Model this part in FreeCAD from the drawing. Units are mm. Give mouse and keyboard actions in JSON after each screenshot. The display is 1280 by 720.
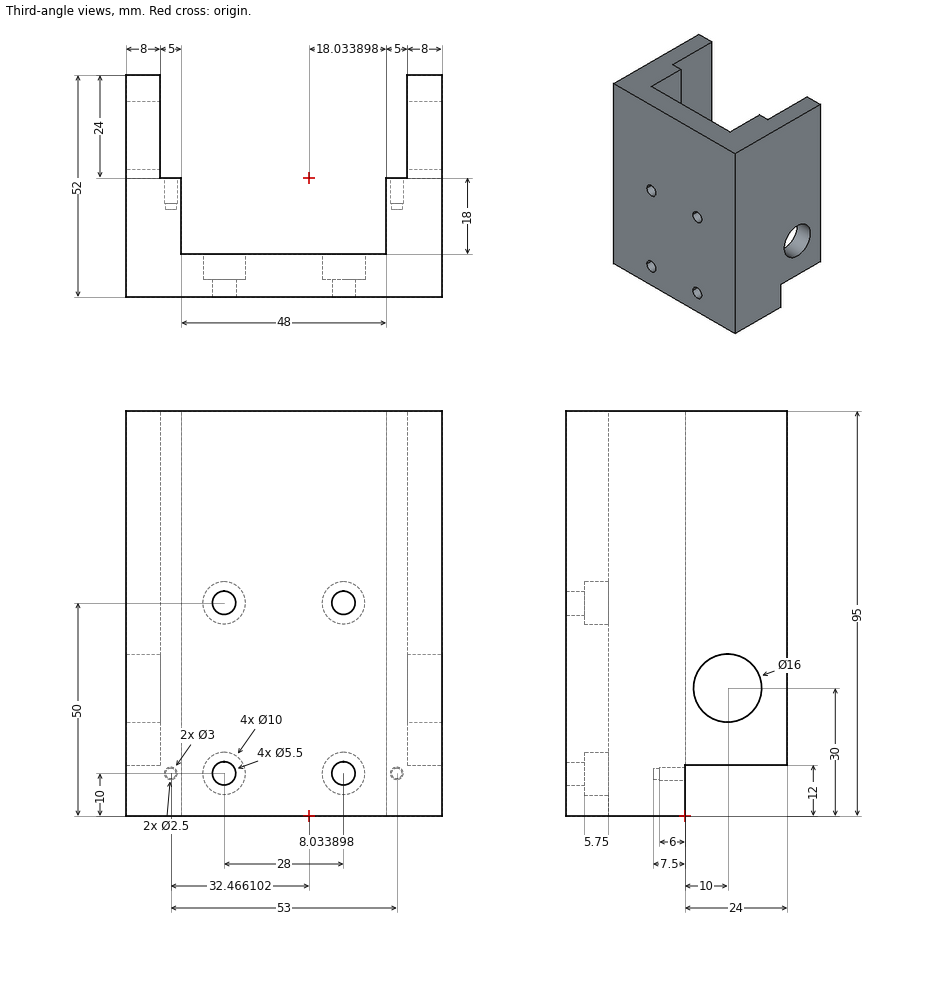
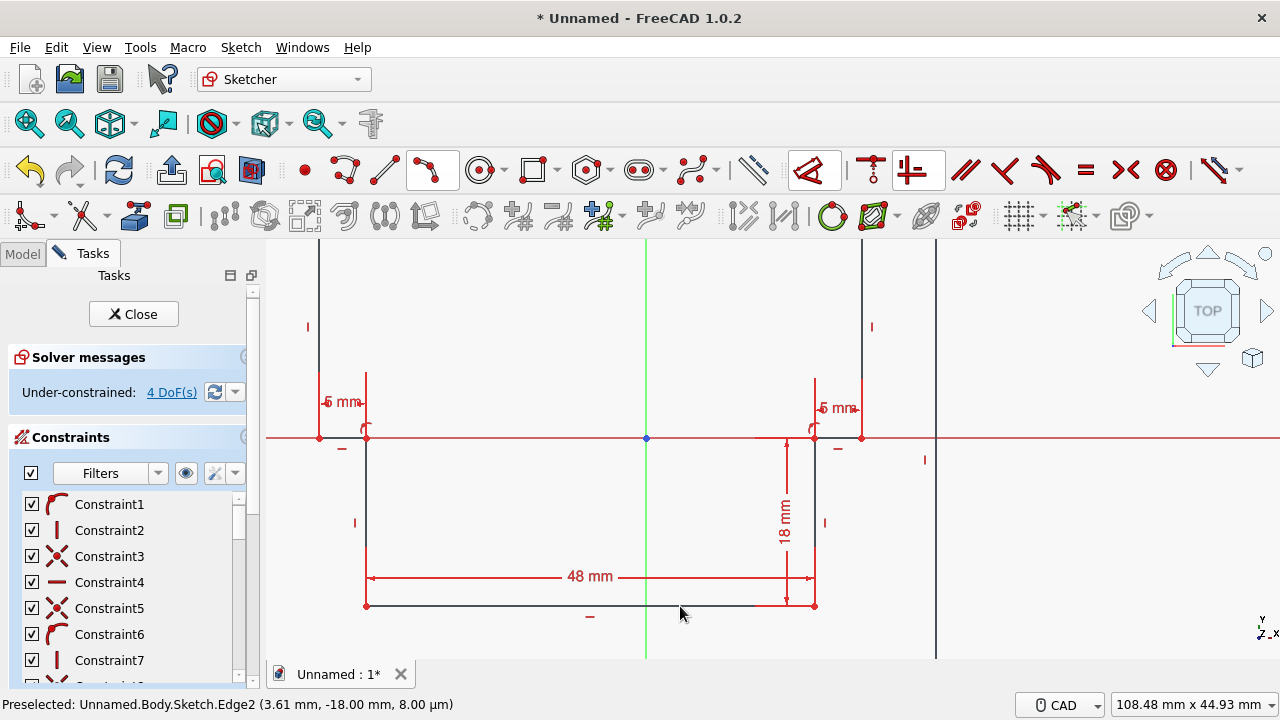
{"action": "left_click", "coordinate": [319, 371]}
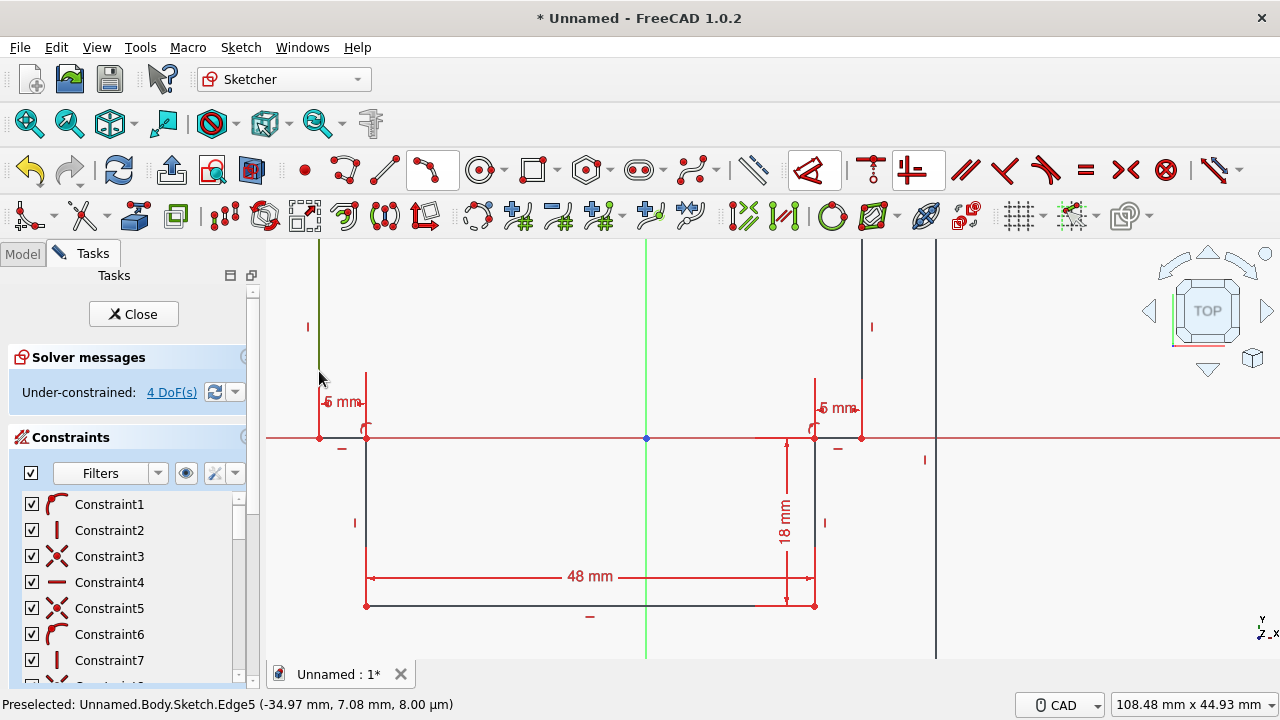
{"action": "key", "text": "i"}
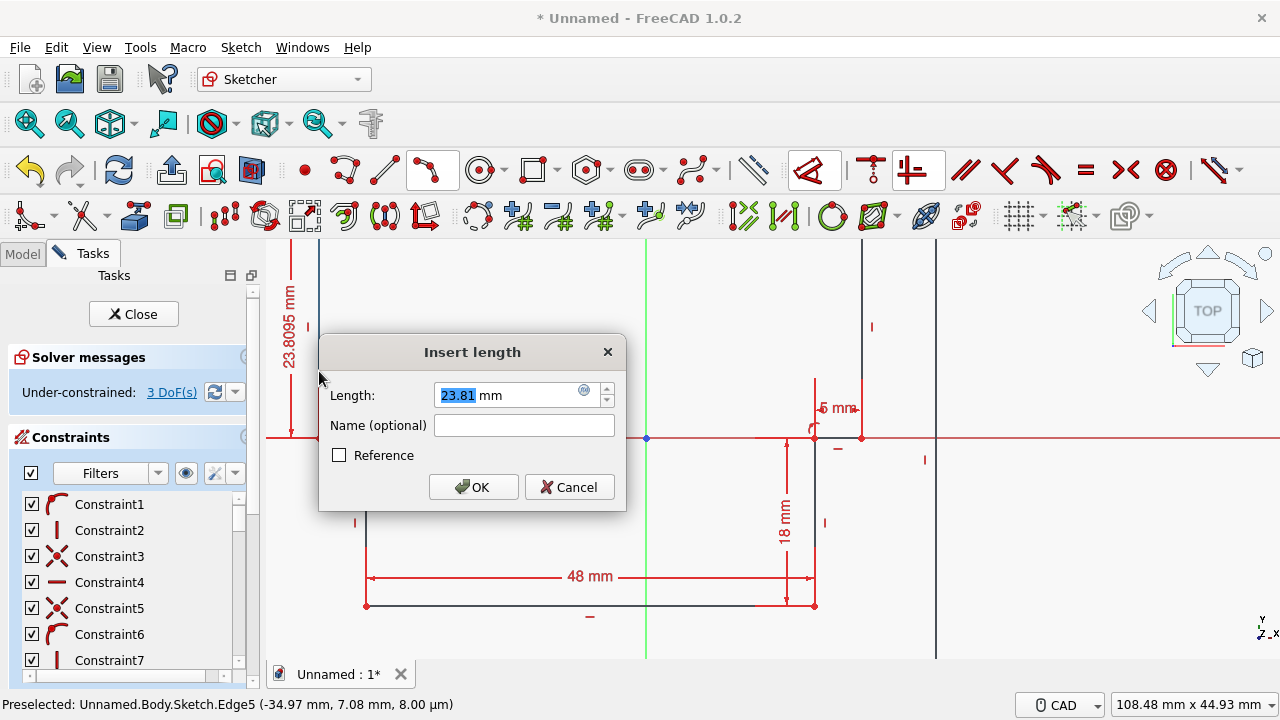
{"action": "type", "text": "24"}
{"action": "key", "text": "Return"}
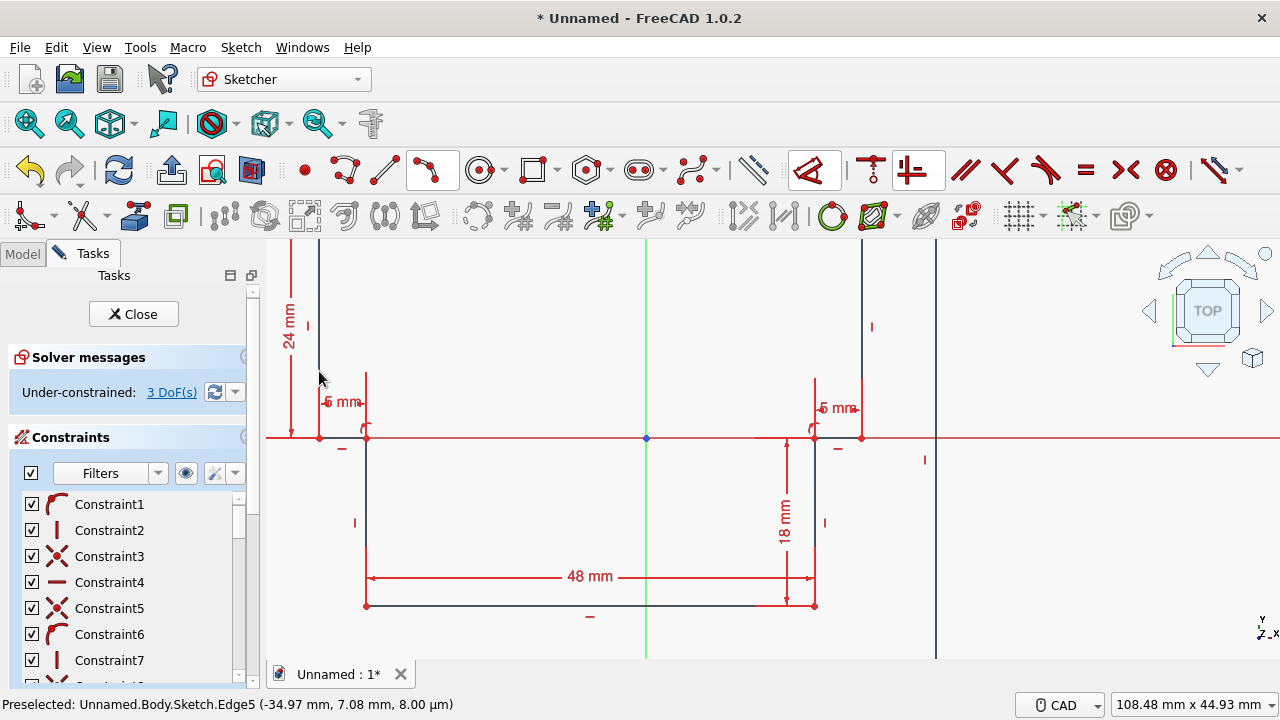
{"action": "scroll", "coordinate": [843, 439], "scroll_direction": "down", "scroll_amount": 3}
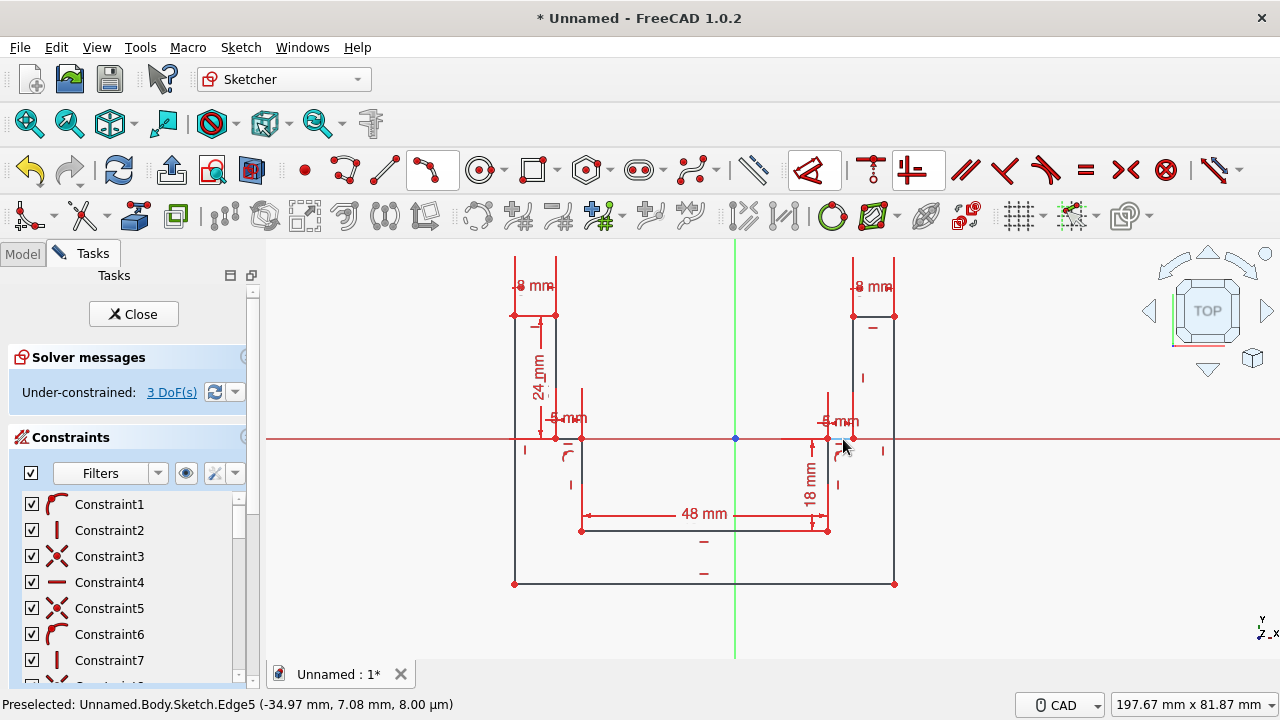
{"action": "left_click", "coordinate": [515, 396]}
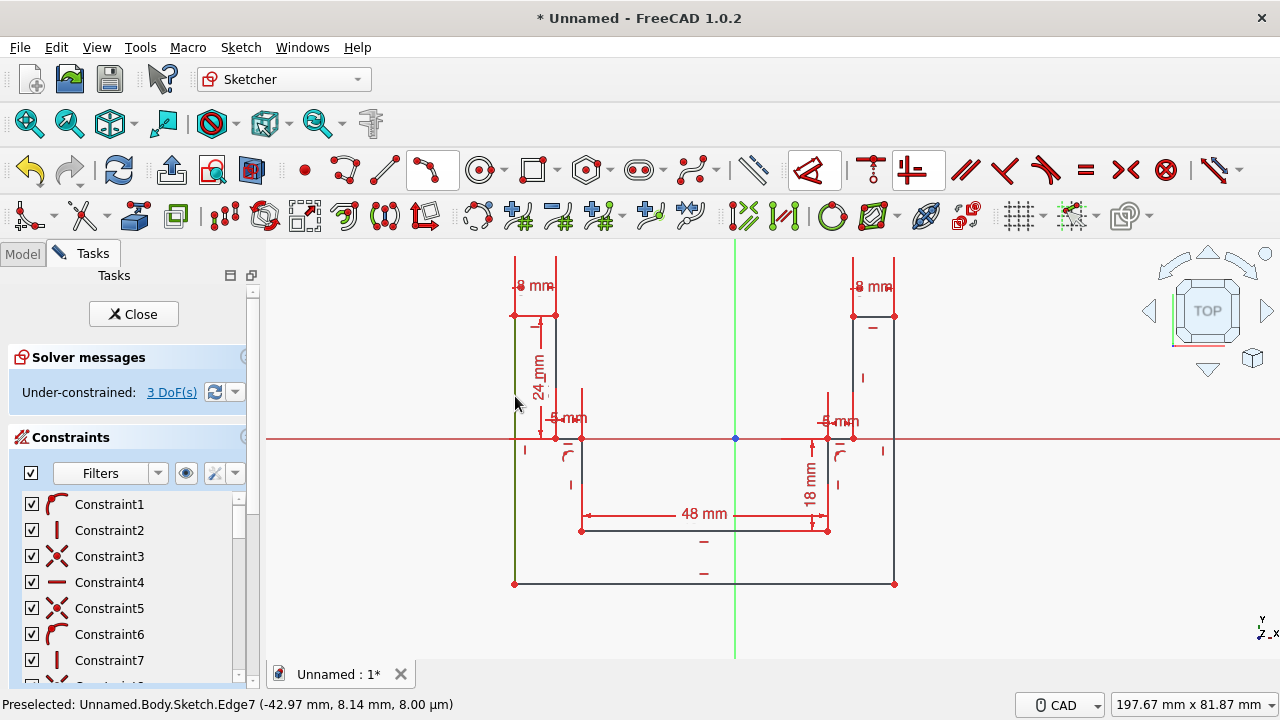
{"action": "key", "text": "i"}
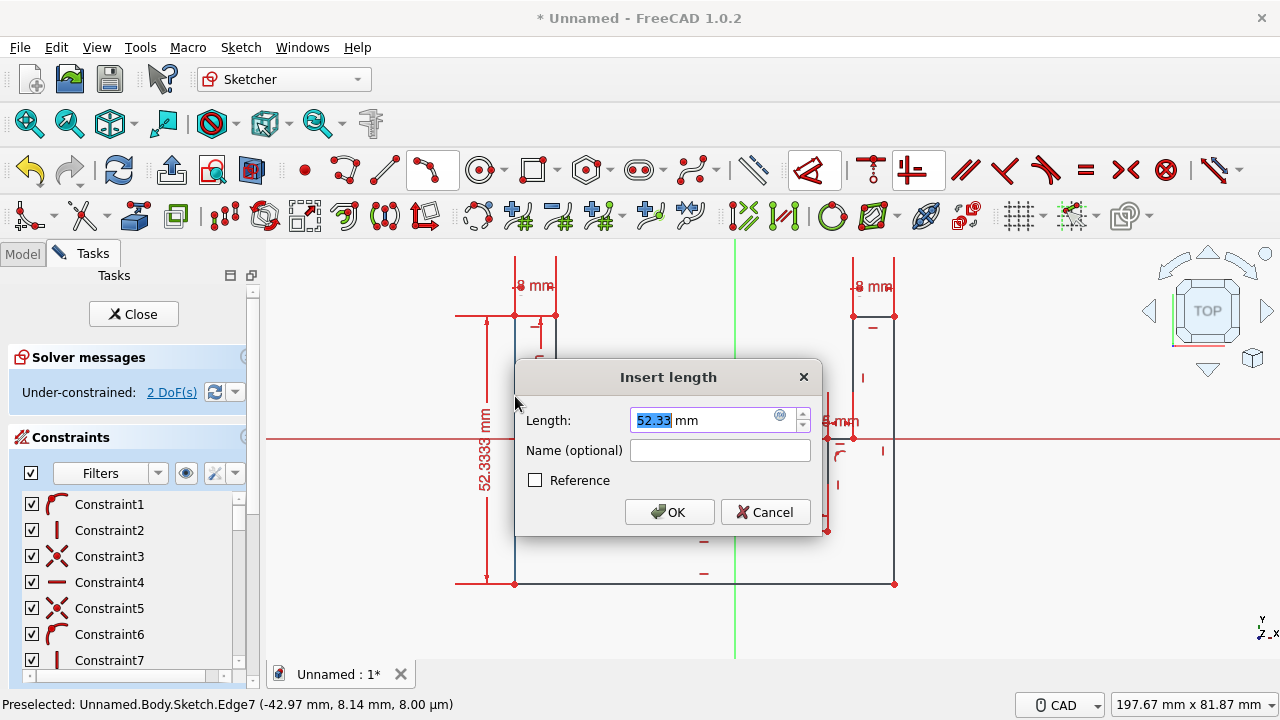
{"action": "type", "text": "52"}
{"action": "key", "text": "Return"}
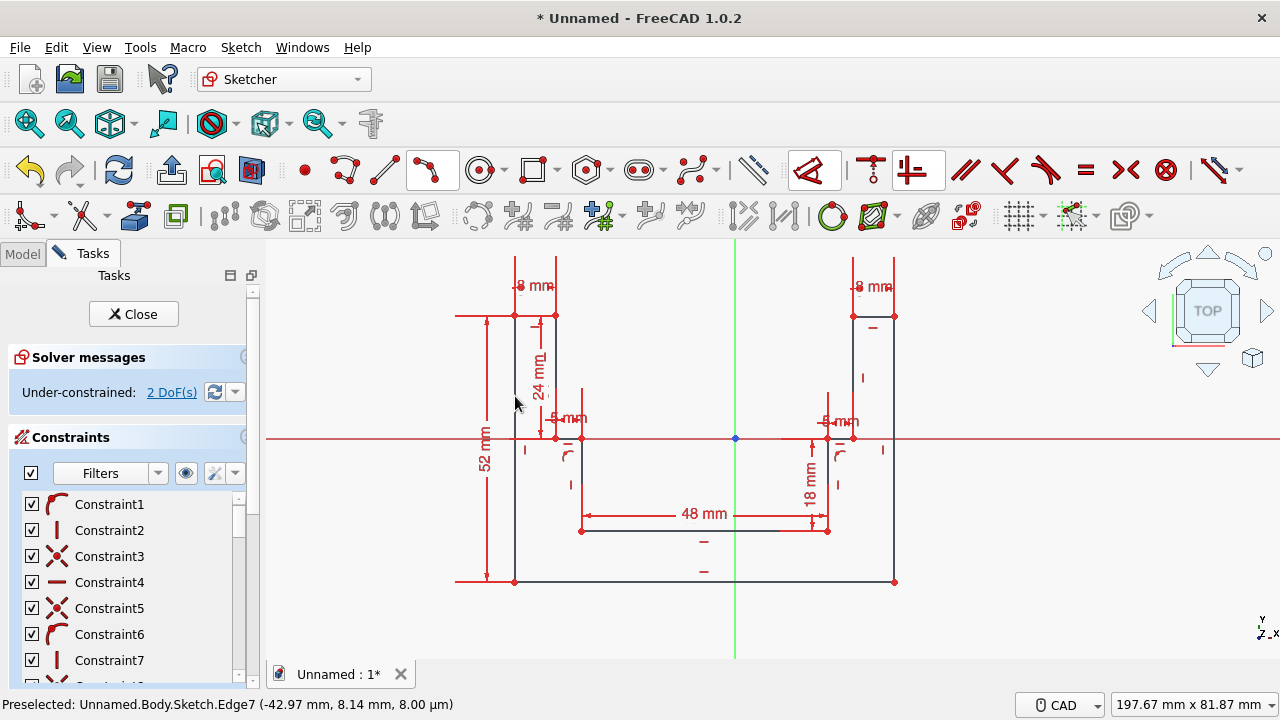
{"action": "left_click", "coordinate": [894, 503]}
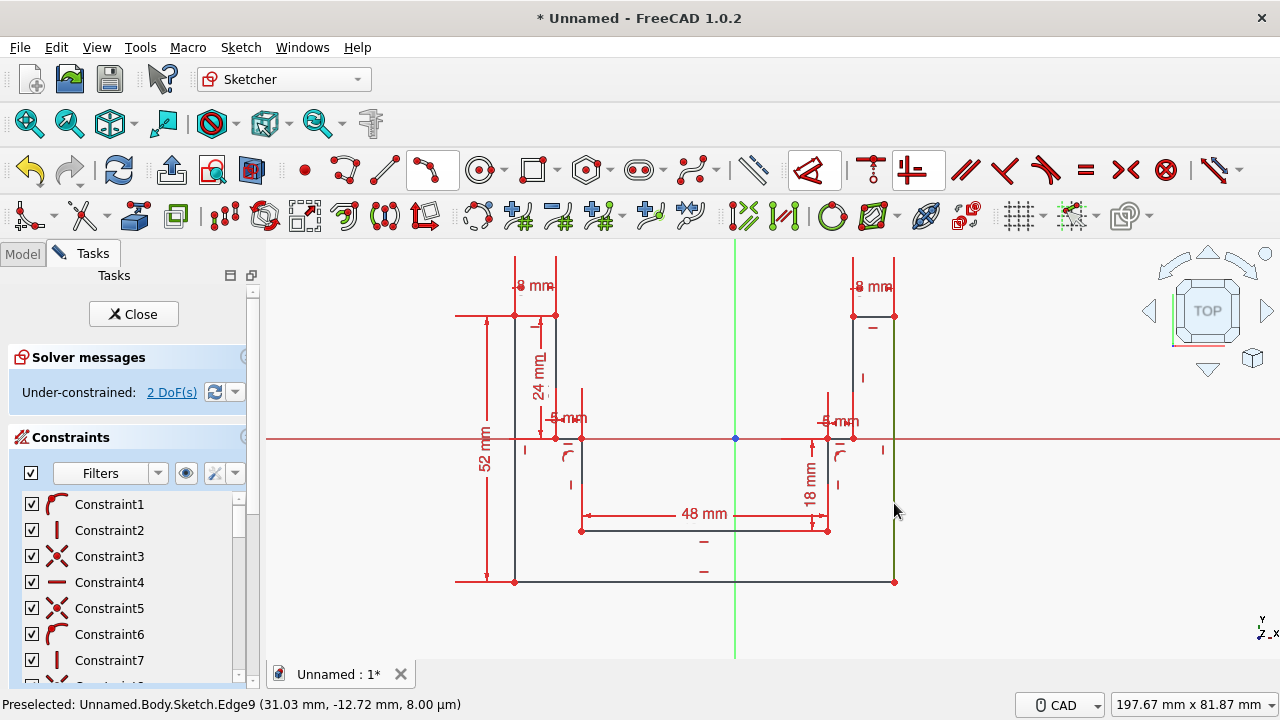
{"action": "left_click", "coordinate": [836, 170]}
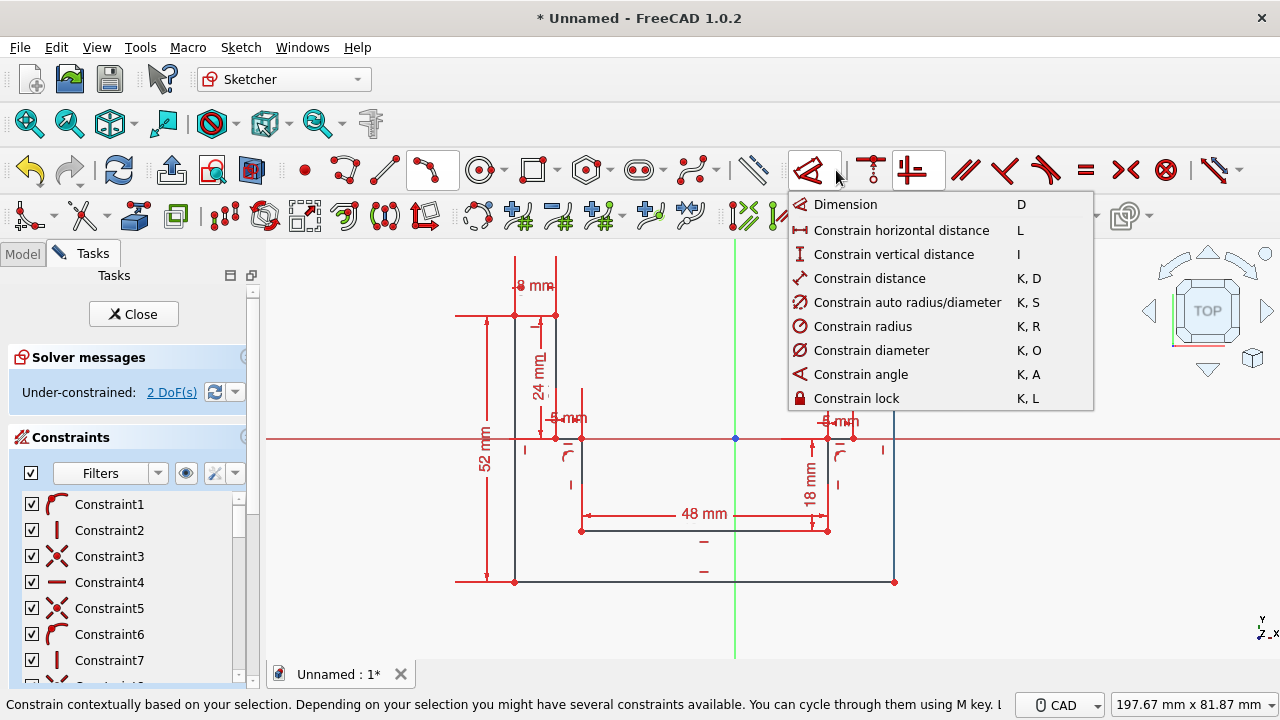
{"action": "left_click", "coordinate": [941, 254]}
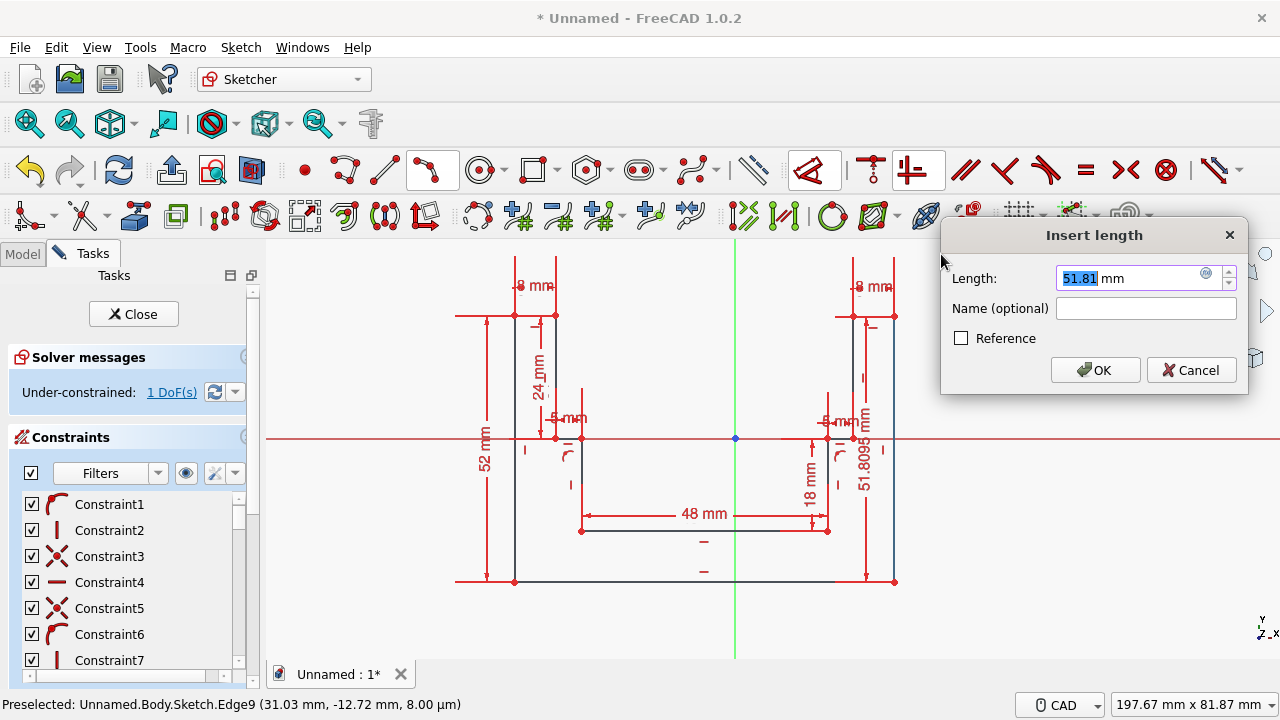
{"action": "type", "text": "52"}
{"action": "key", "text": "Return"}